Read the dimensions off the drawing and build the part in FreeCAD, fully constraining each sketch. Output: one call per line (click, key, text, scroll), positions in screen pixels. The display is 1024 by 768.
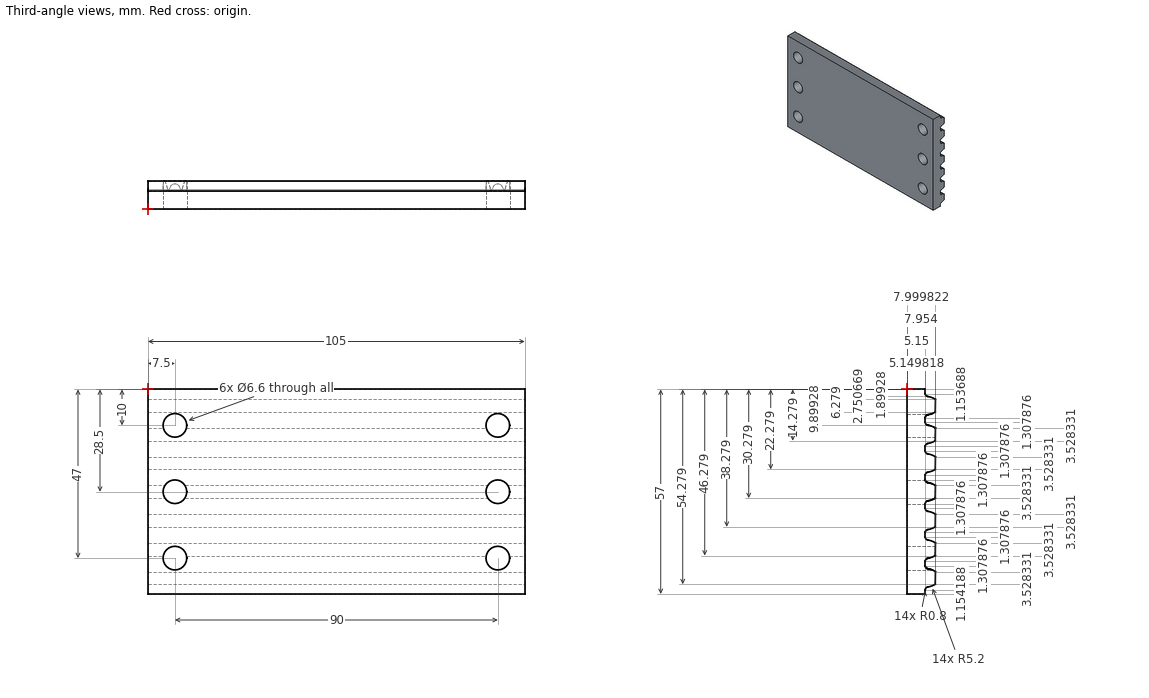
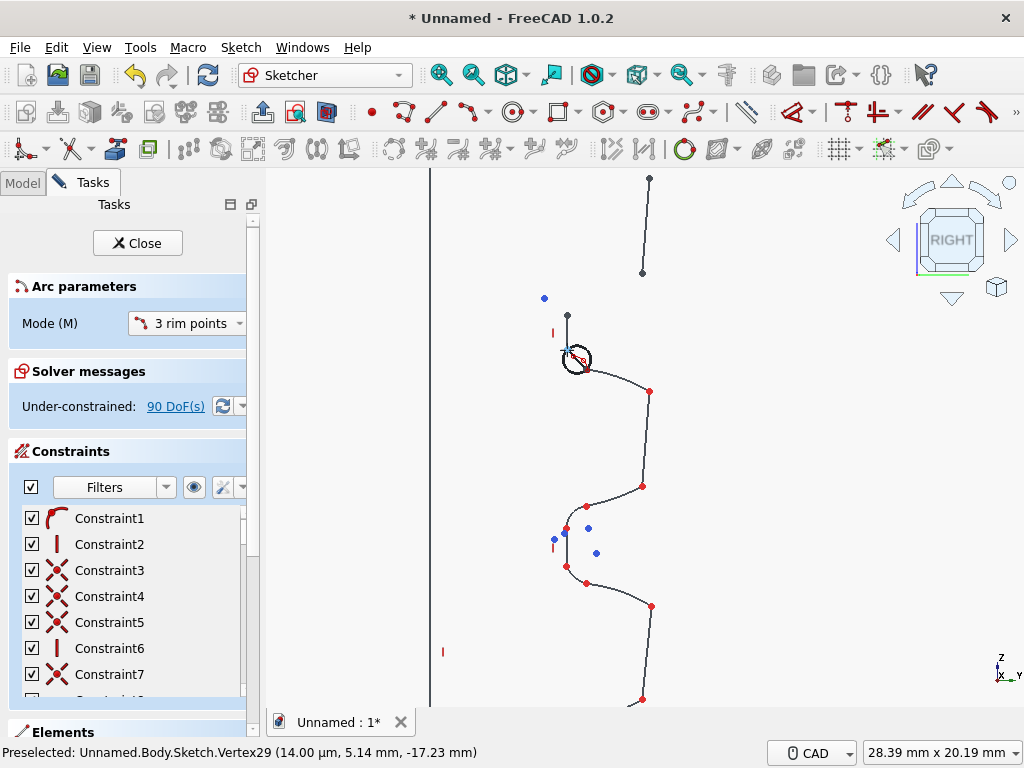
scroll(573, 362, up, 6)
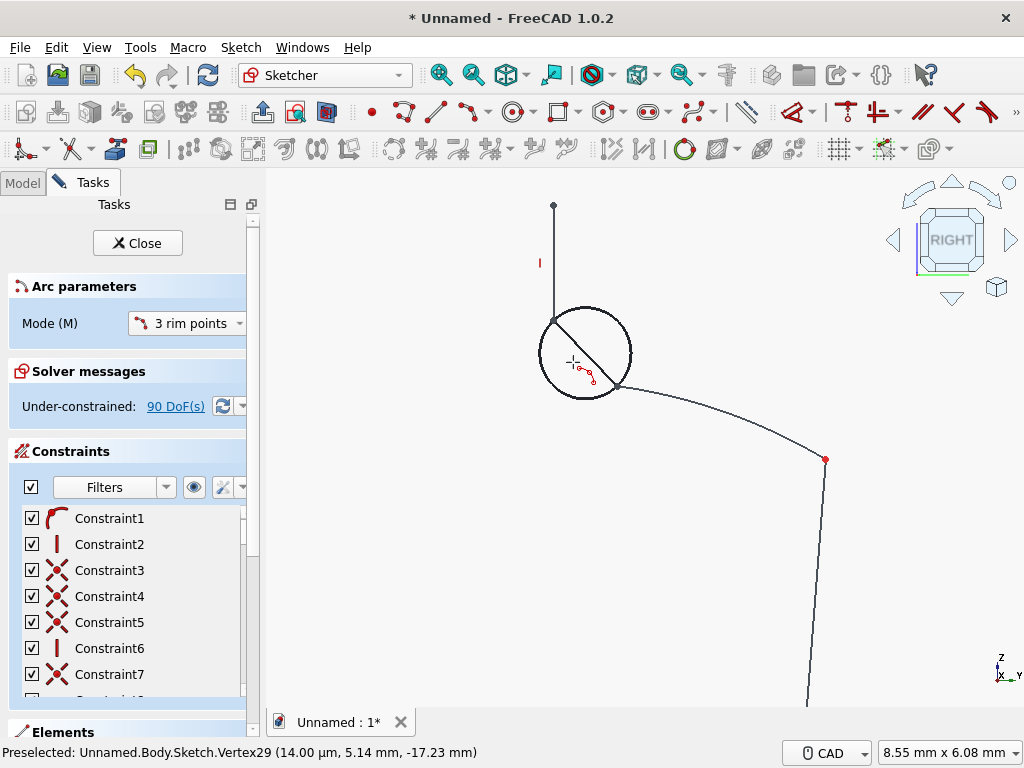
click(572, 360)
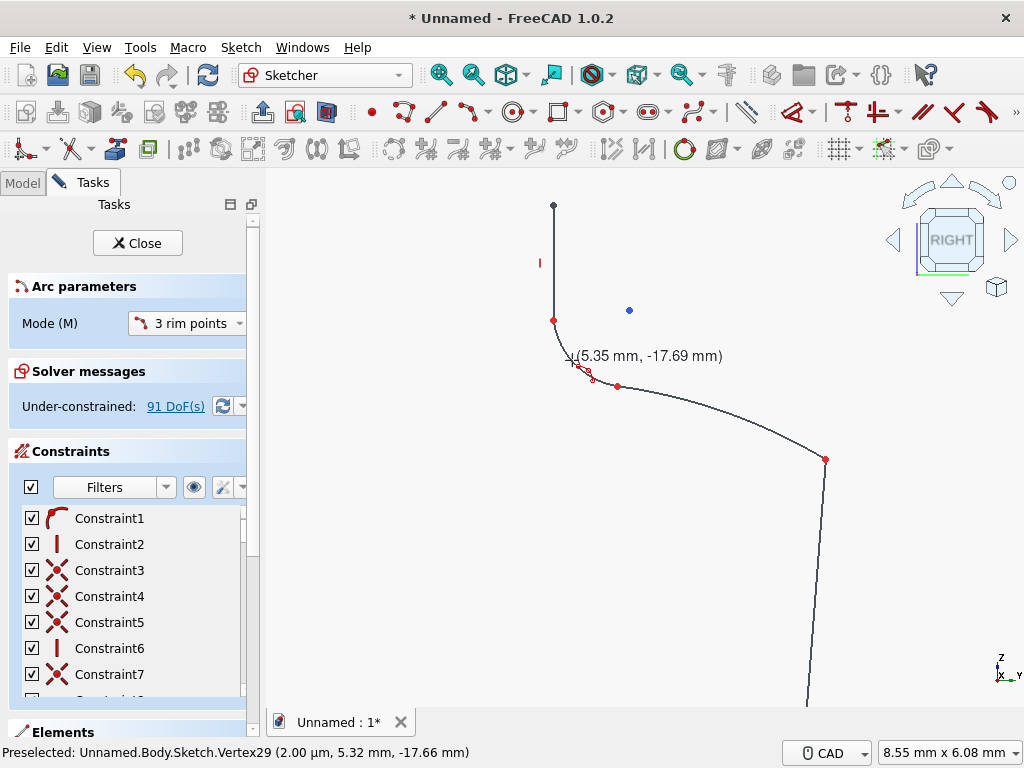
scroll(586, 367, down, 13)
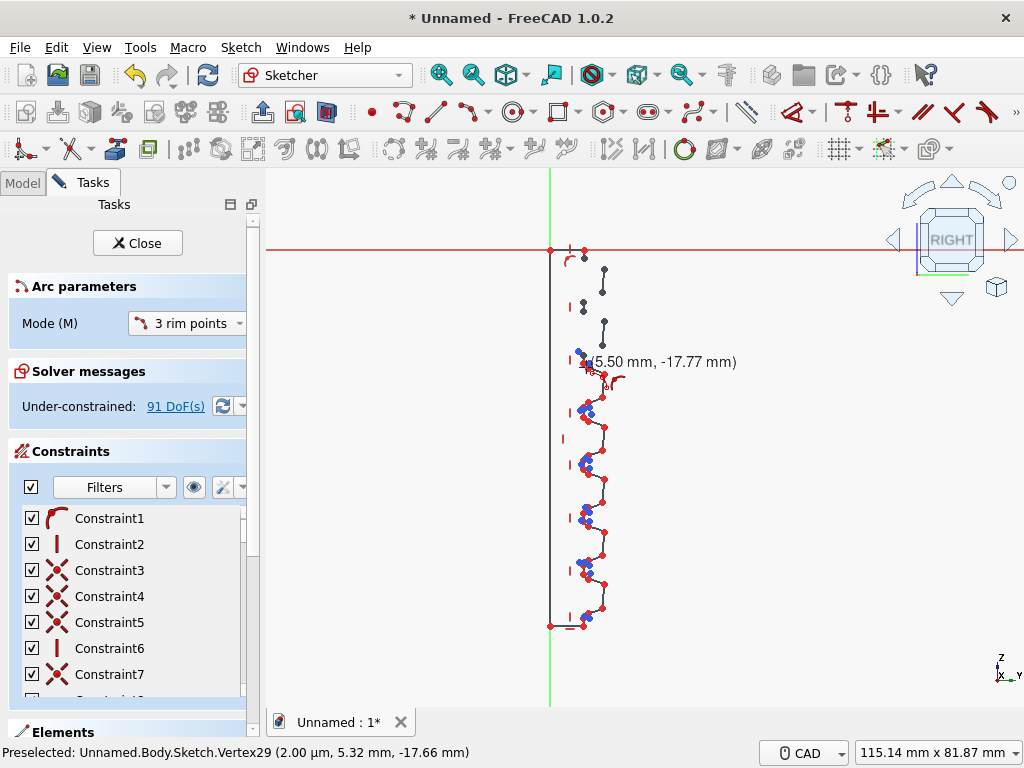
scroll(584, 355, up, 7)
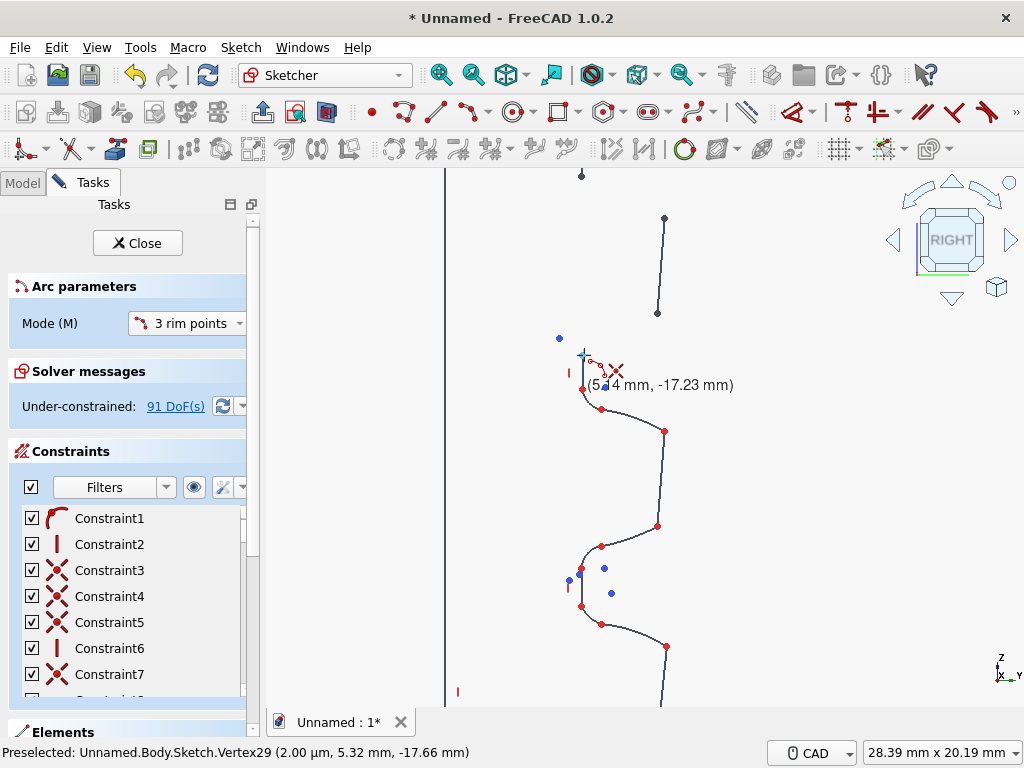
click(583, 355)
click(601, 332)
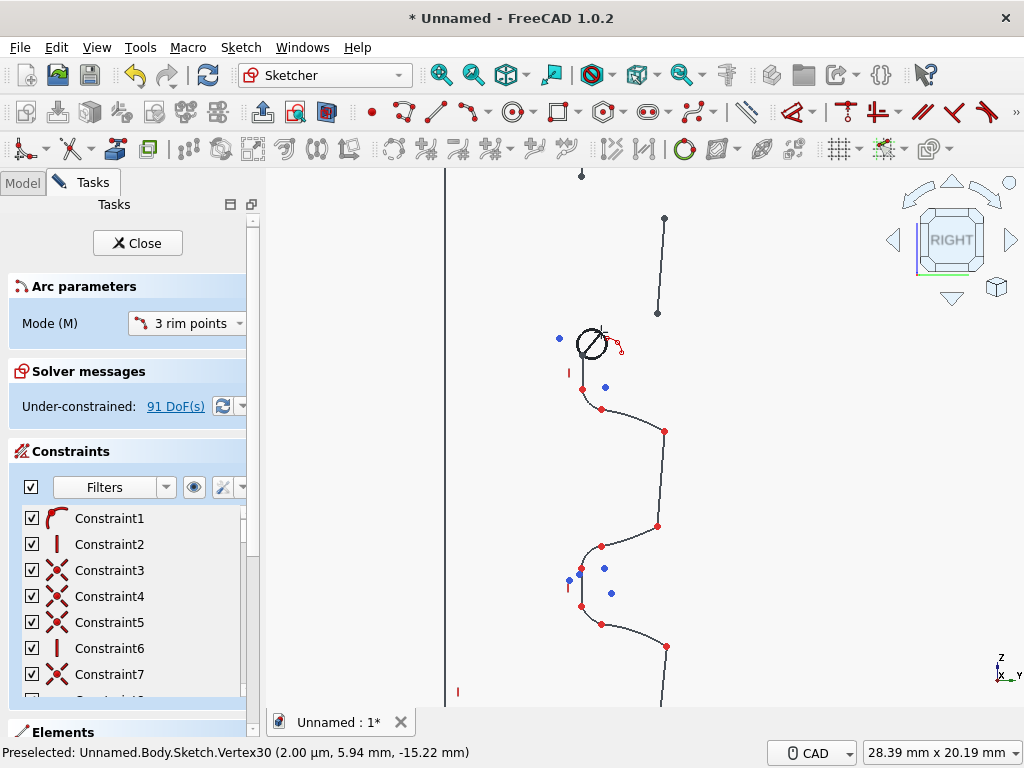
scroll(588, 339, up, 6)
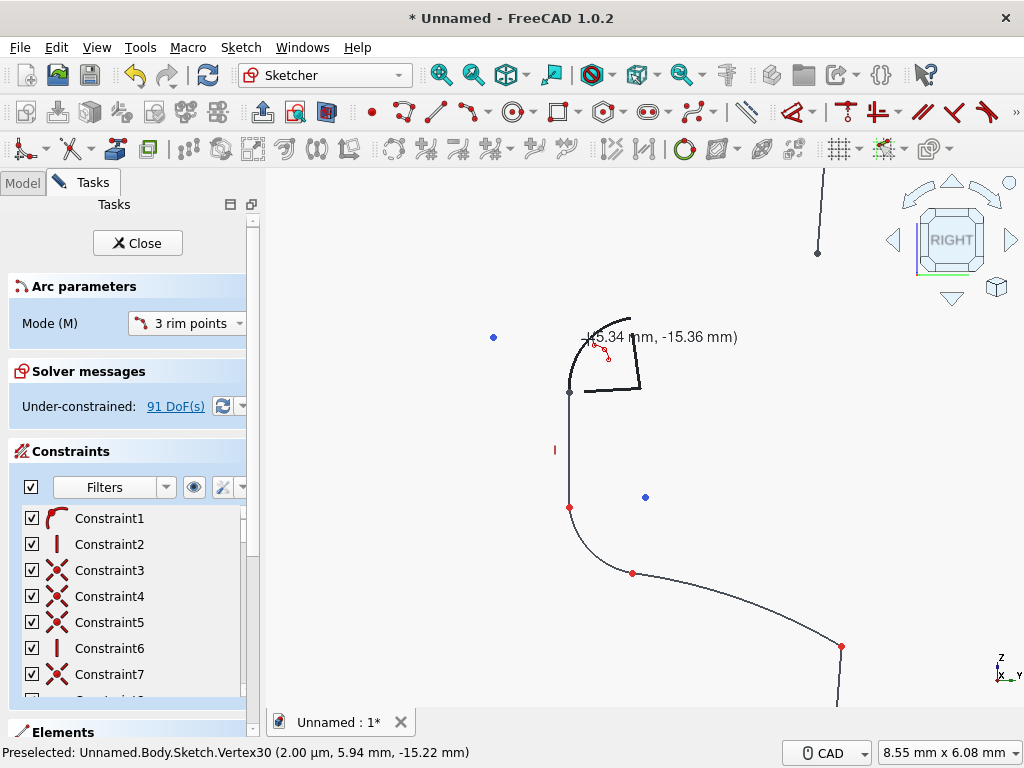
click(588, 338)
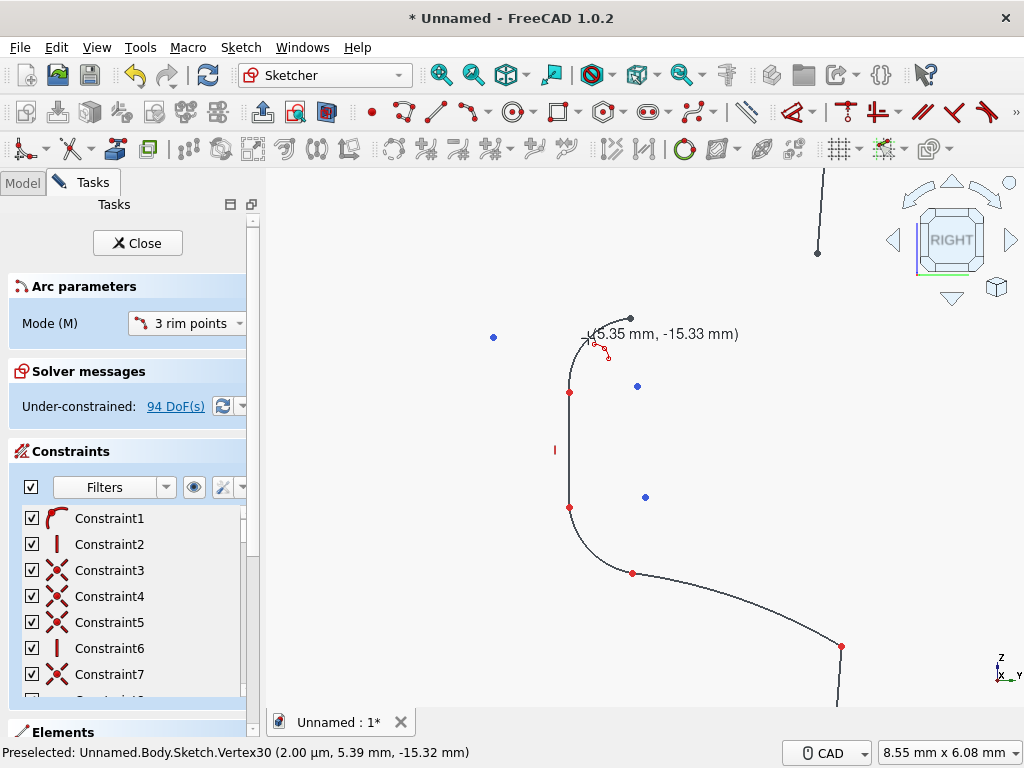
scroll(585, 352, down, 13)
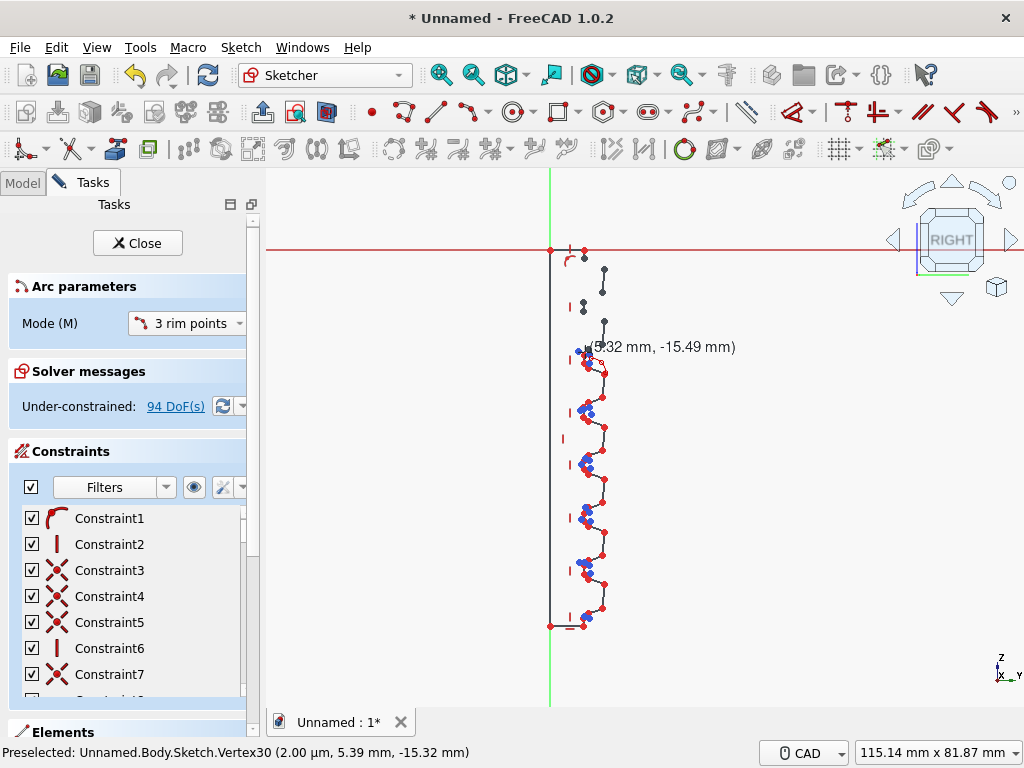
scroll(589, 350, up, 6)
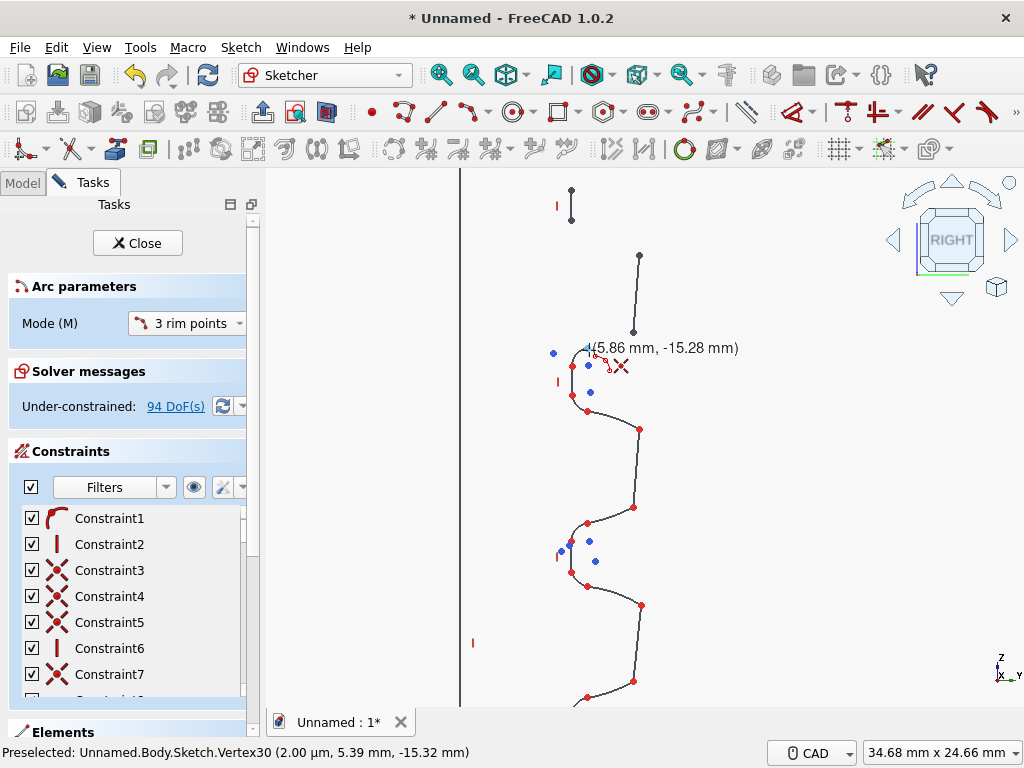
click(587, 349)
click(633, 333)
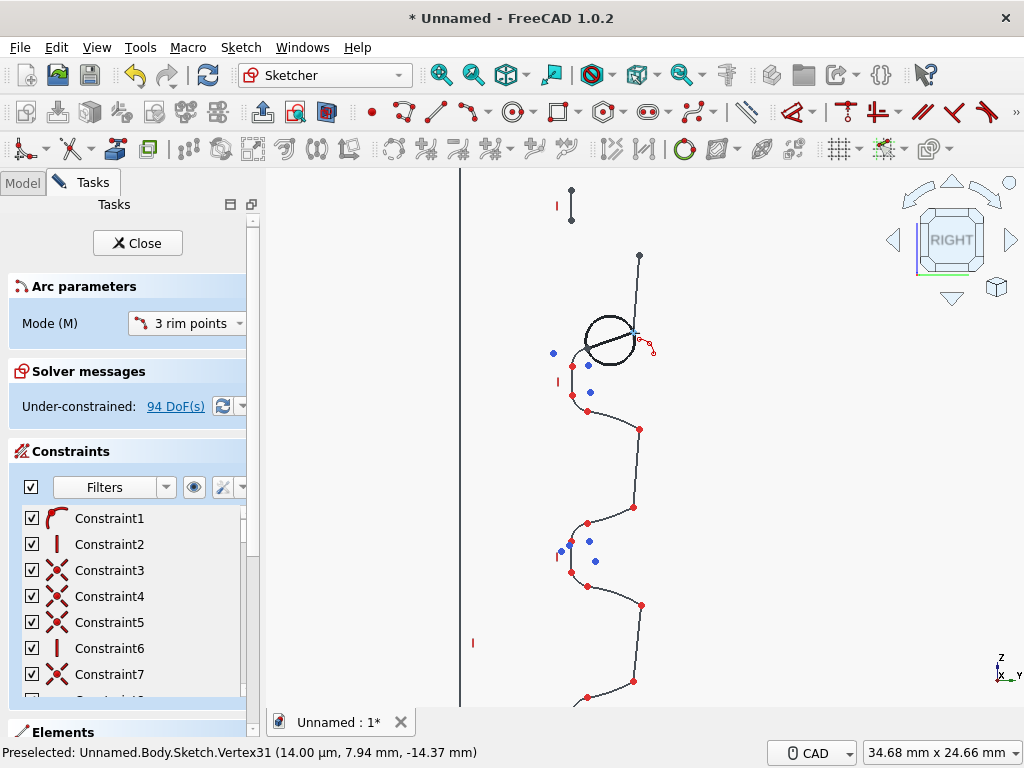
scroll(612, 342, up, 9)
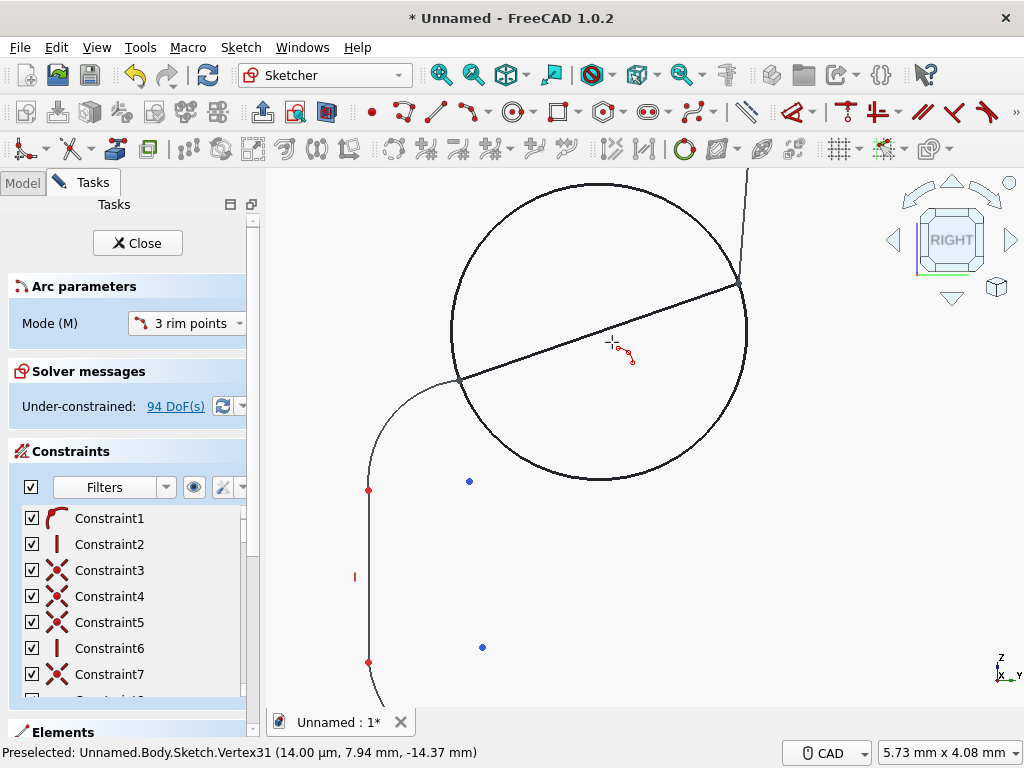
click(607, 338)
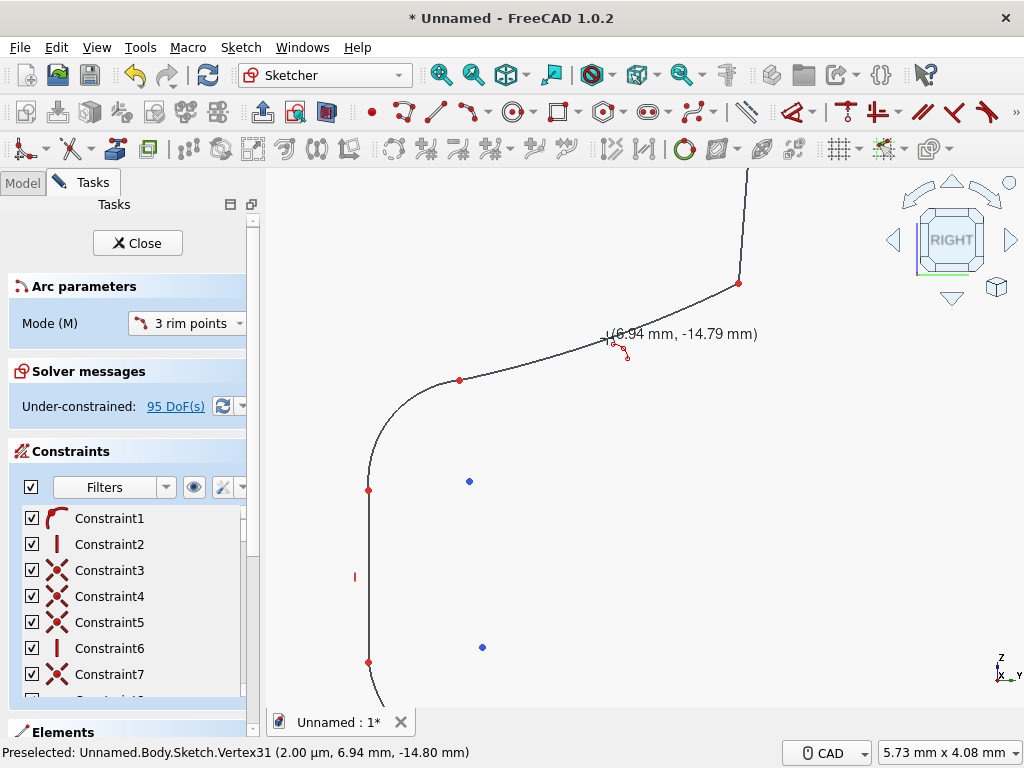
scroll(595, 348, down, 15)